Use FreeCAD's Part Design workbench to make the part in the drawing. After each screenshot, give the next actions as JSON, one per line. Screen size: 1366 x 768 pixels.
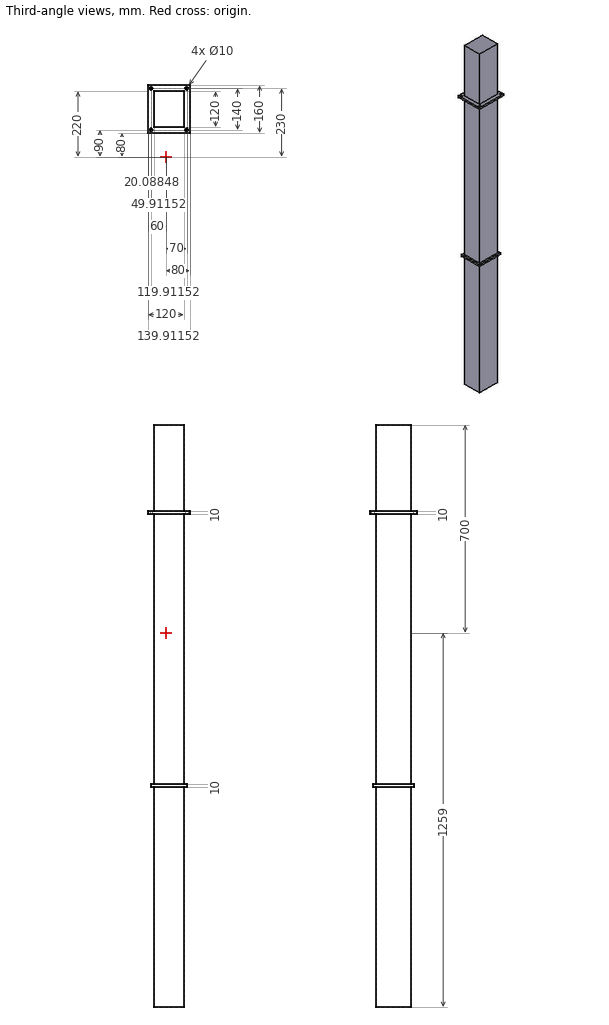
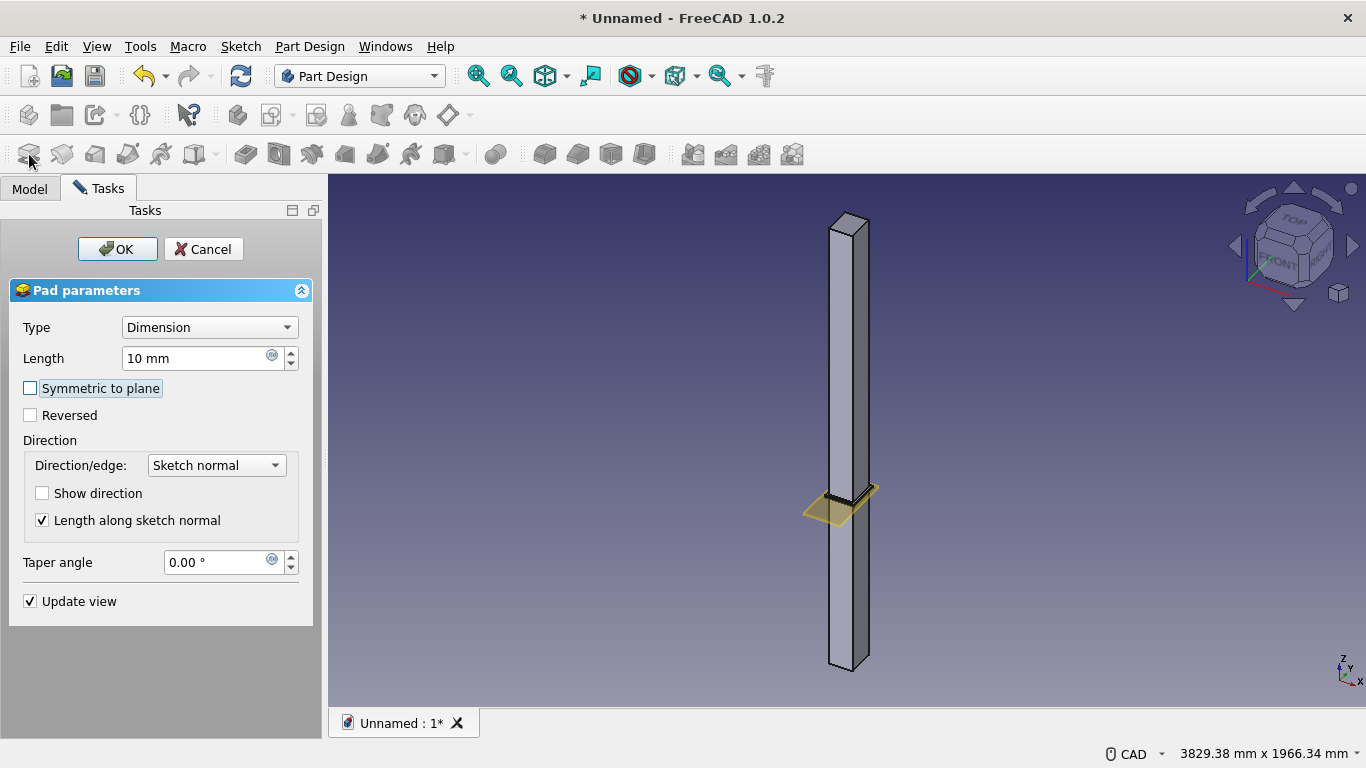
{"action": "left_click", "coordinate": [31, 415]}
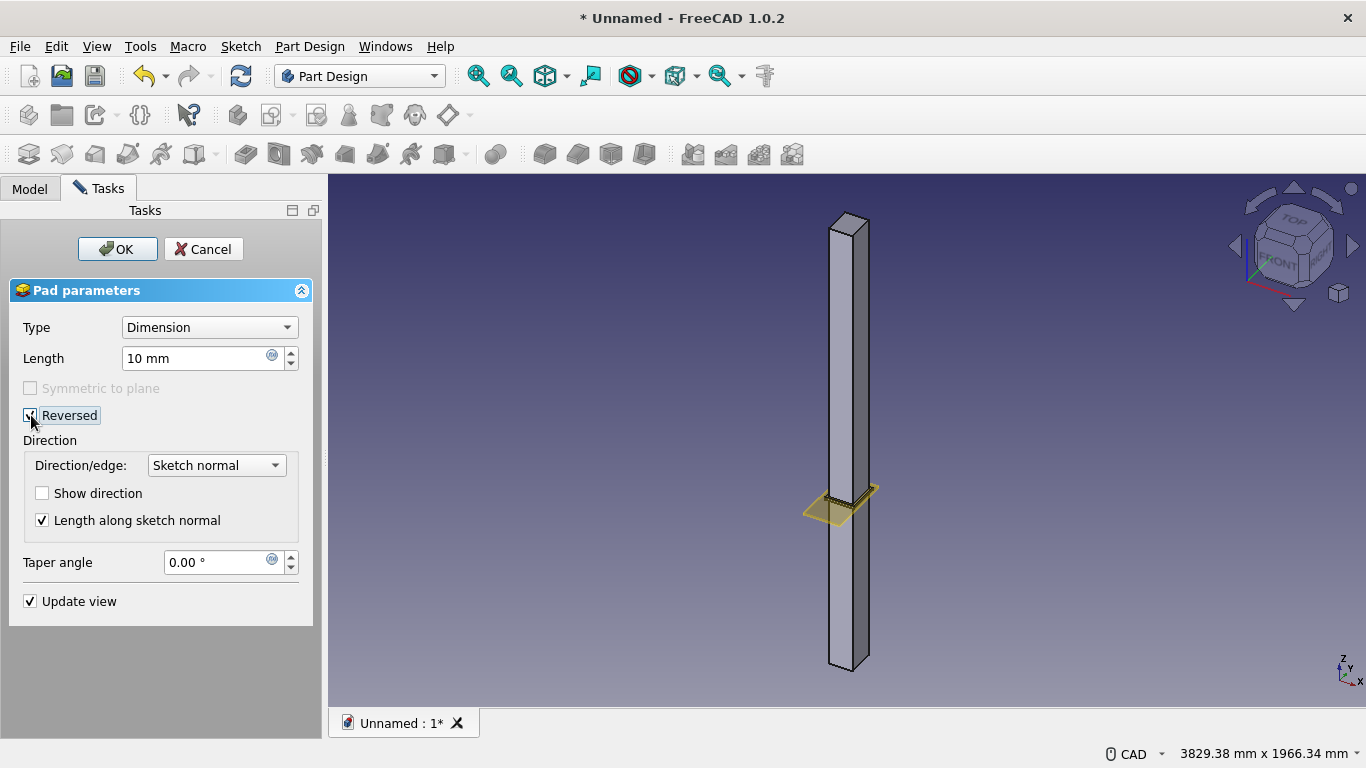
{"action": "left_click", "coordinate": [118, 249]}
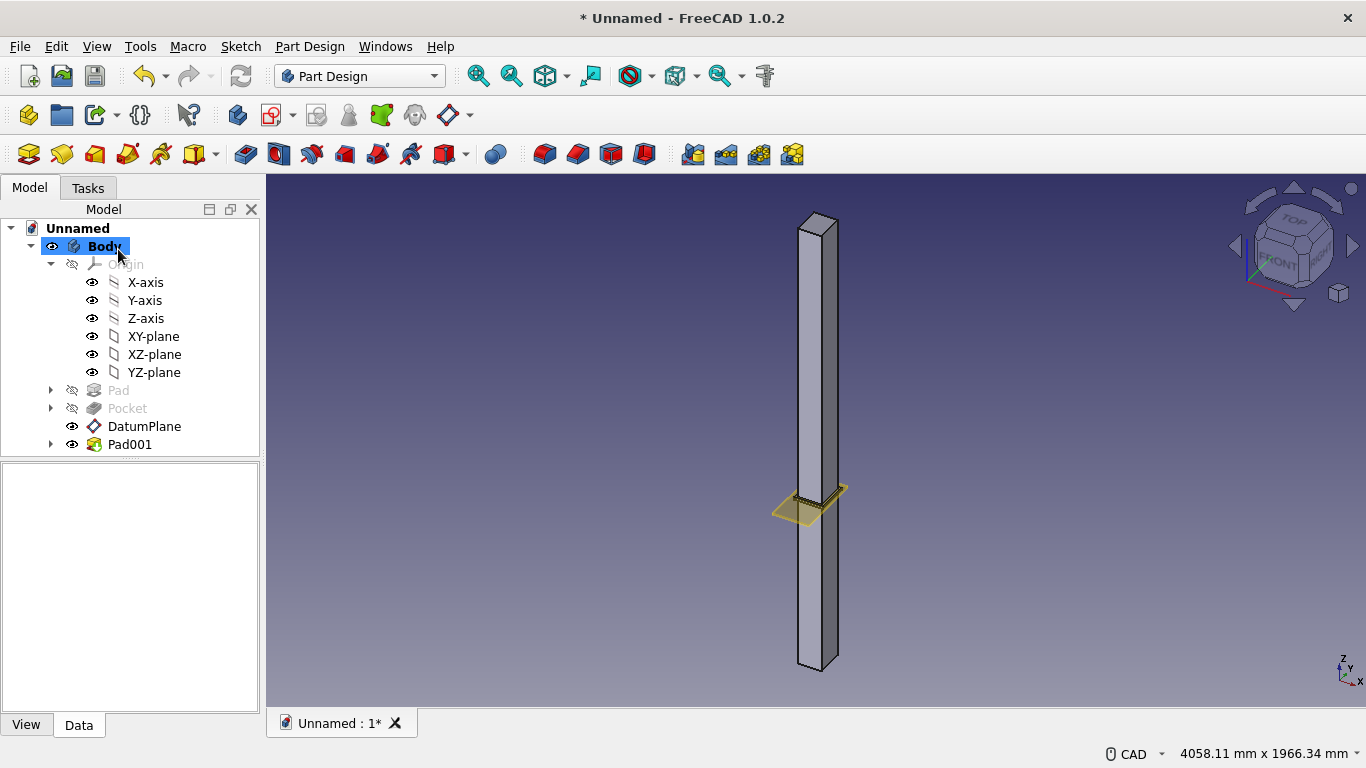
{"action": "left_click", "coordinate": [117, 426]}
{"action": "key", "text": "space"}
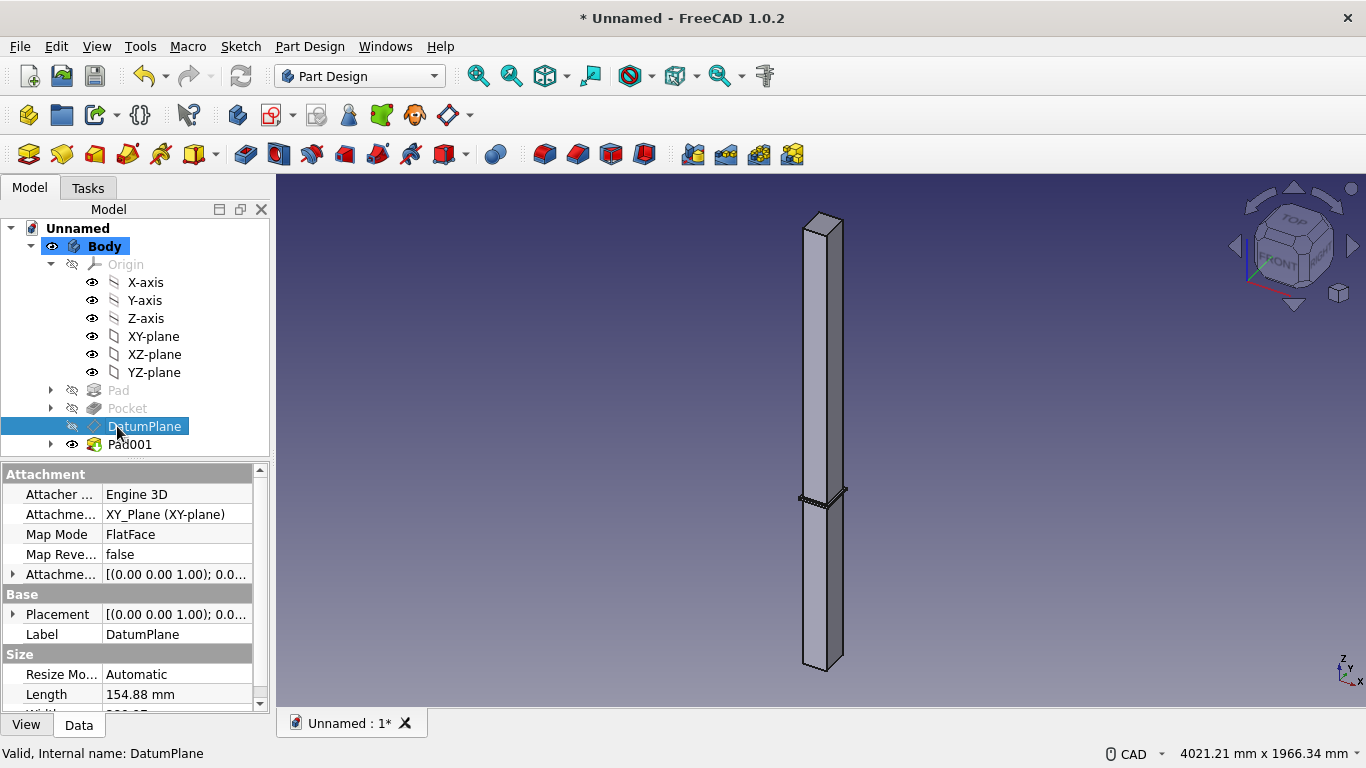
{"action": "left_click", "coordinate": [137, 336]}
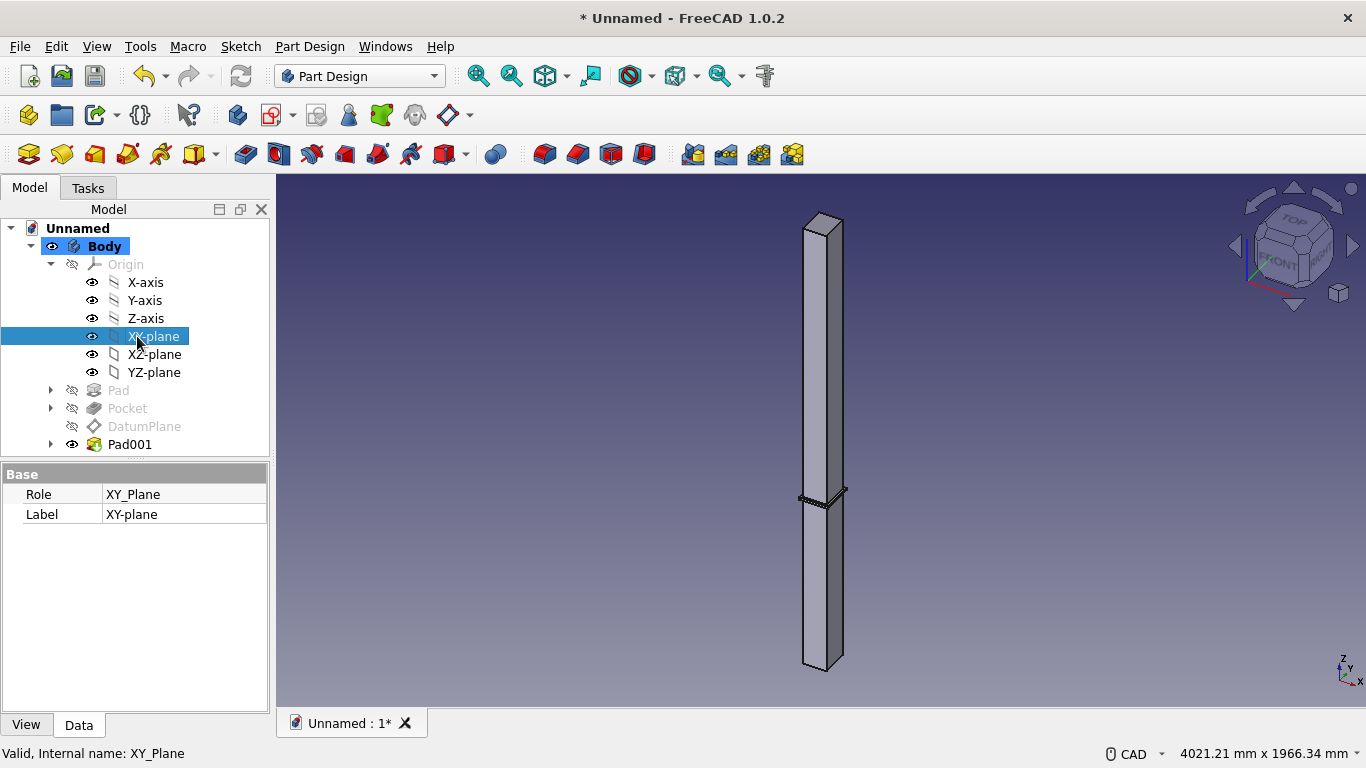
{"action": "left_click", "coordinate": [448, 116]}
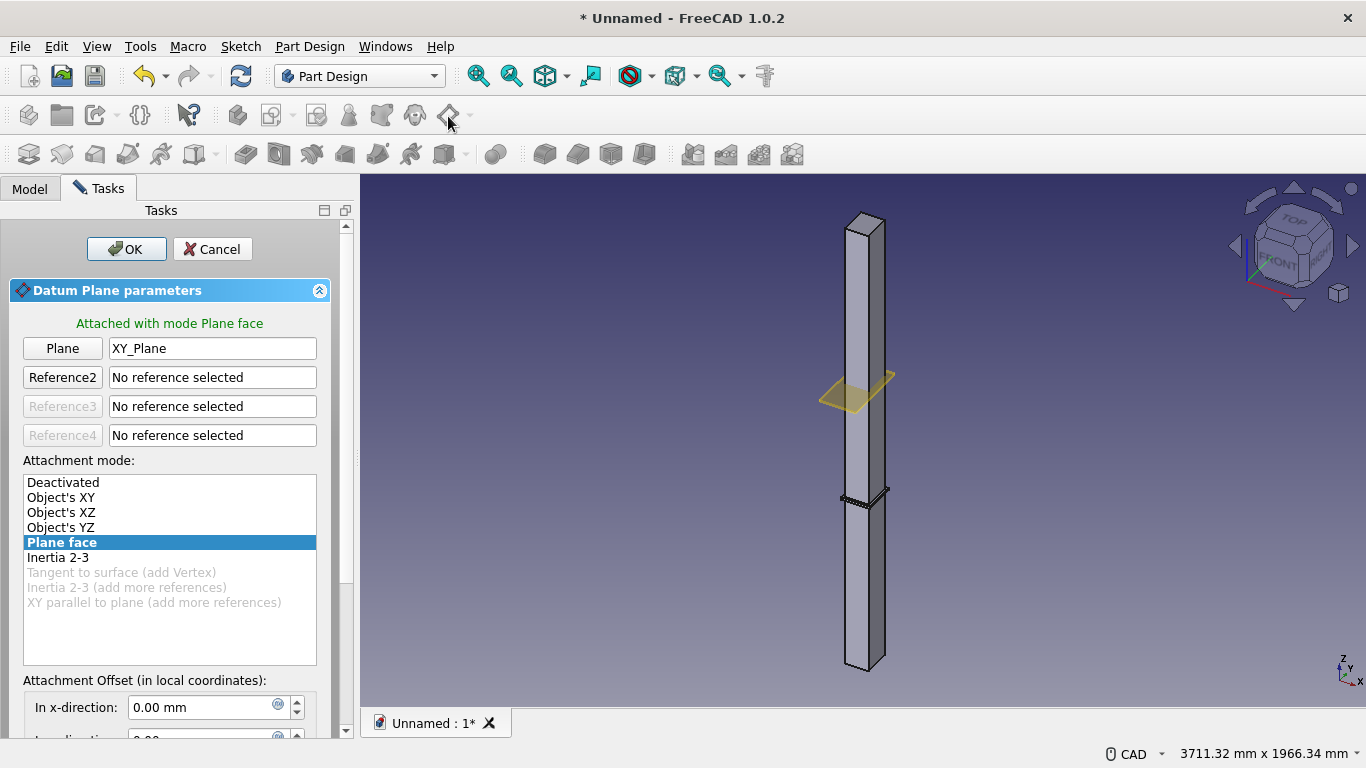
{"action": "scroll", "coordinate": [346, 479], "scroll_direction": "down", "scroll_amount": 2}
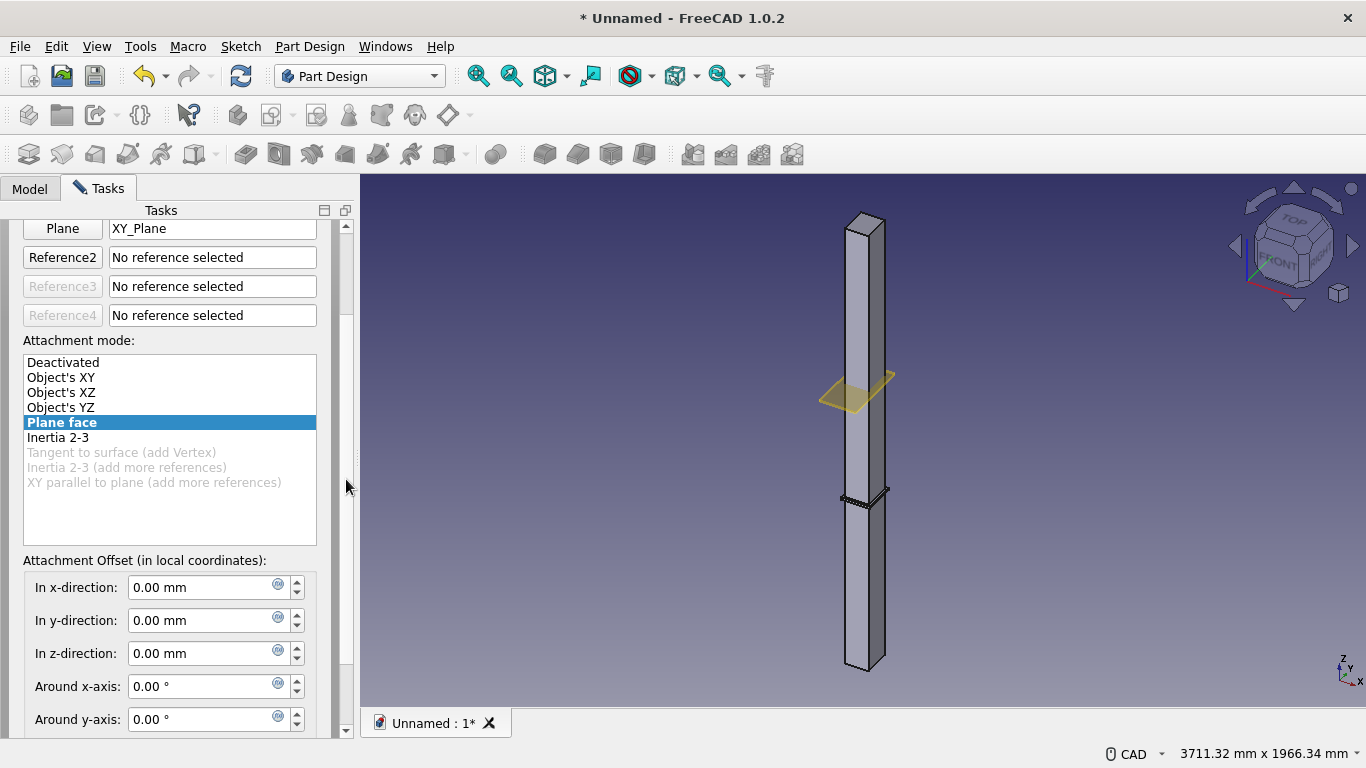
{"action": "triple_click", "coordinate": [210, 654]}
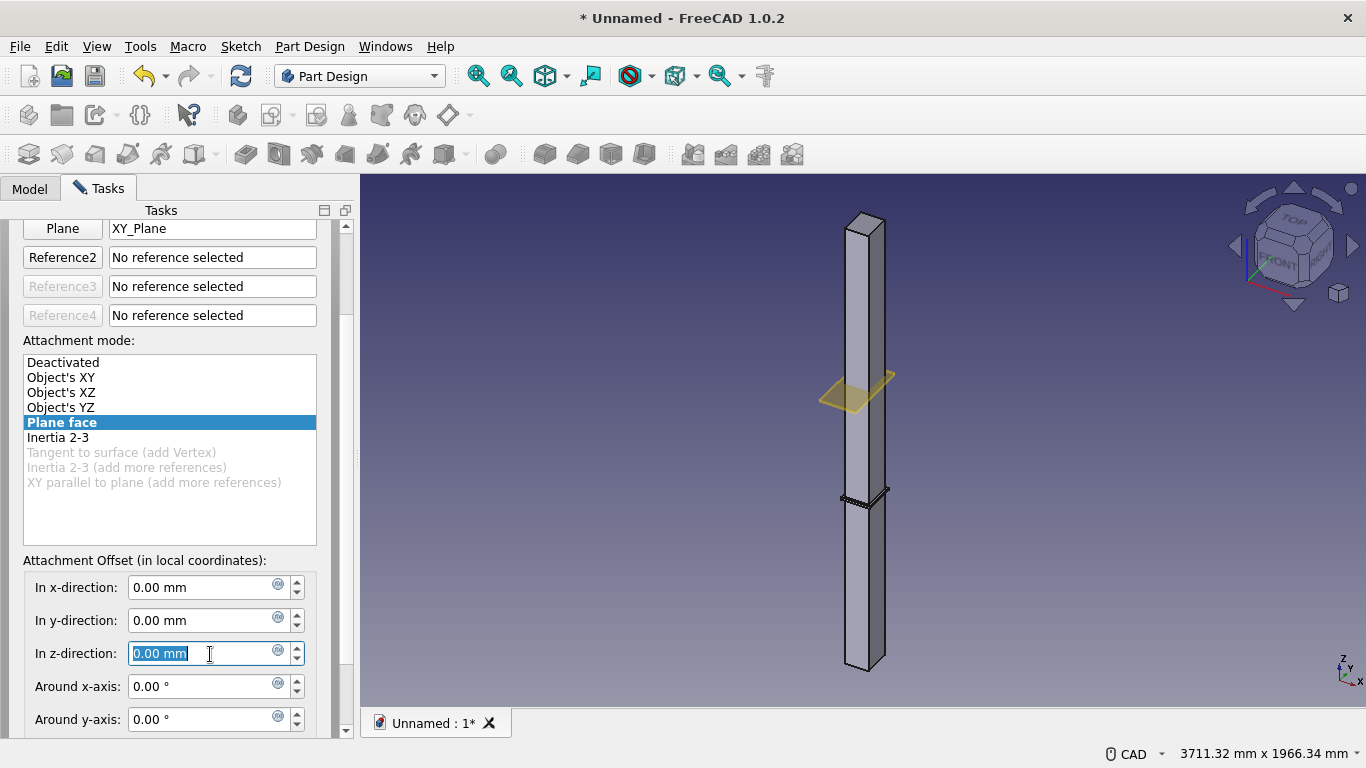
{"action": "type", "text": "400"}
{"action": "key", "text": "Tab"}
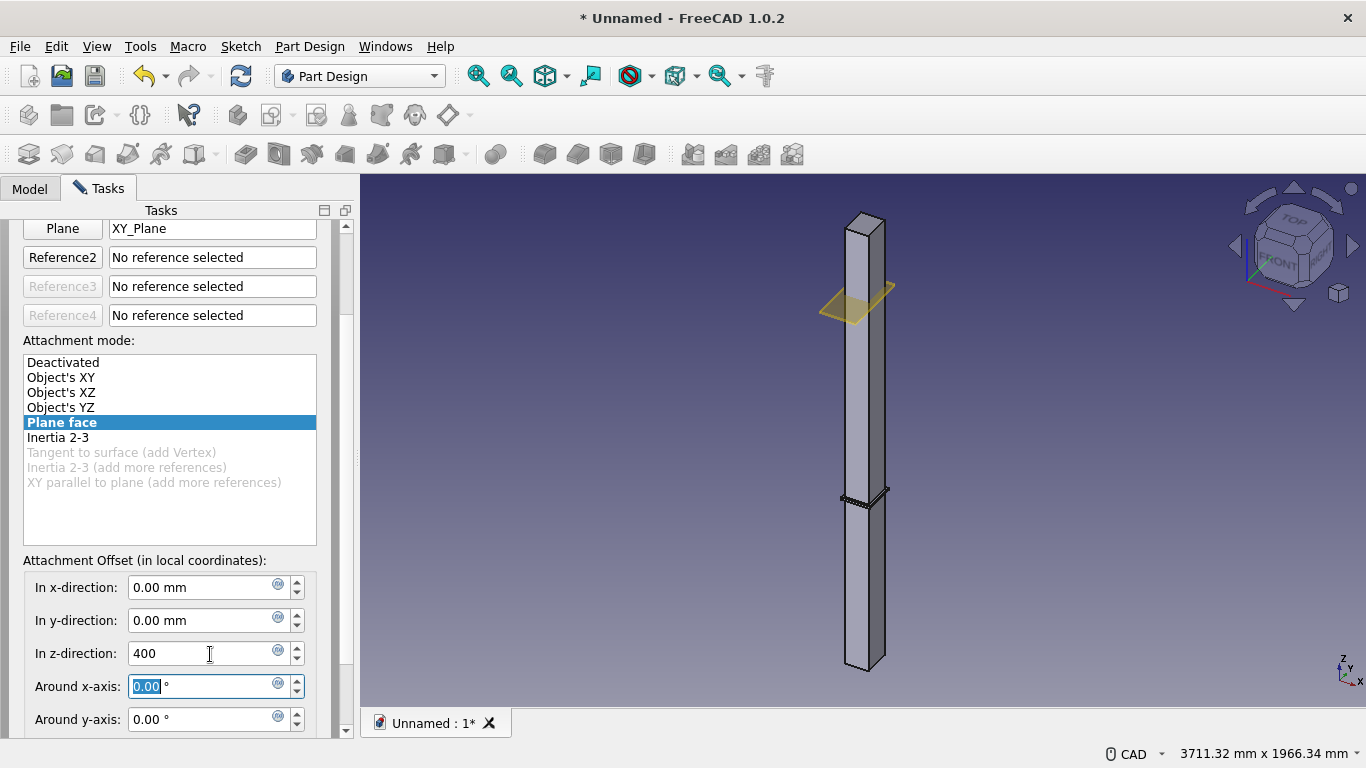
{"action": "scroll", "coordinate": [346, 479], "scroll_direction": "up", "scroll_amount": 3}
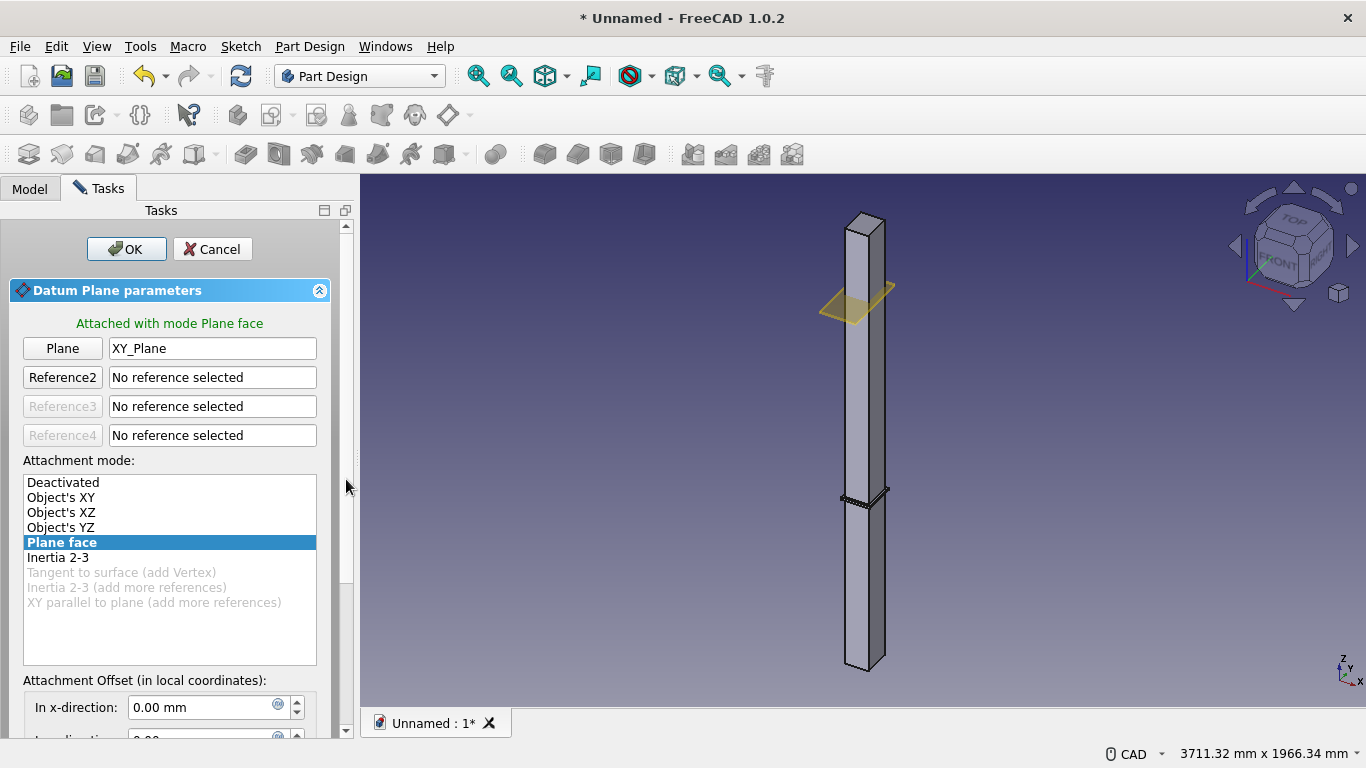
{"action": "left_click", "coordinate": [127, 249]}